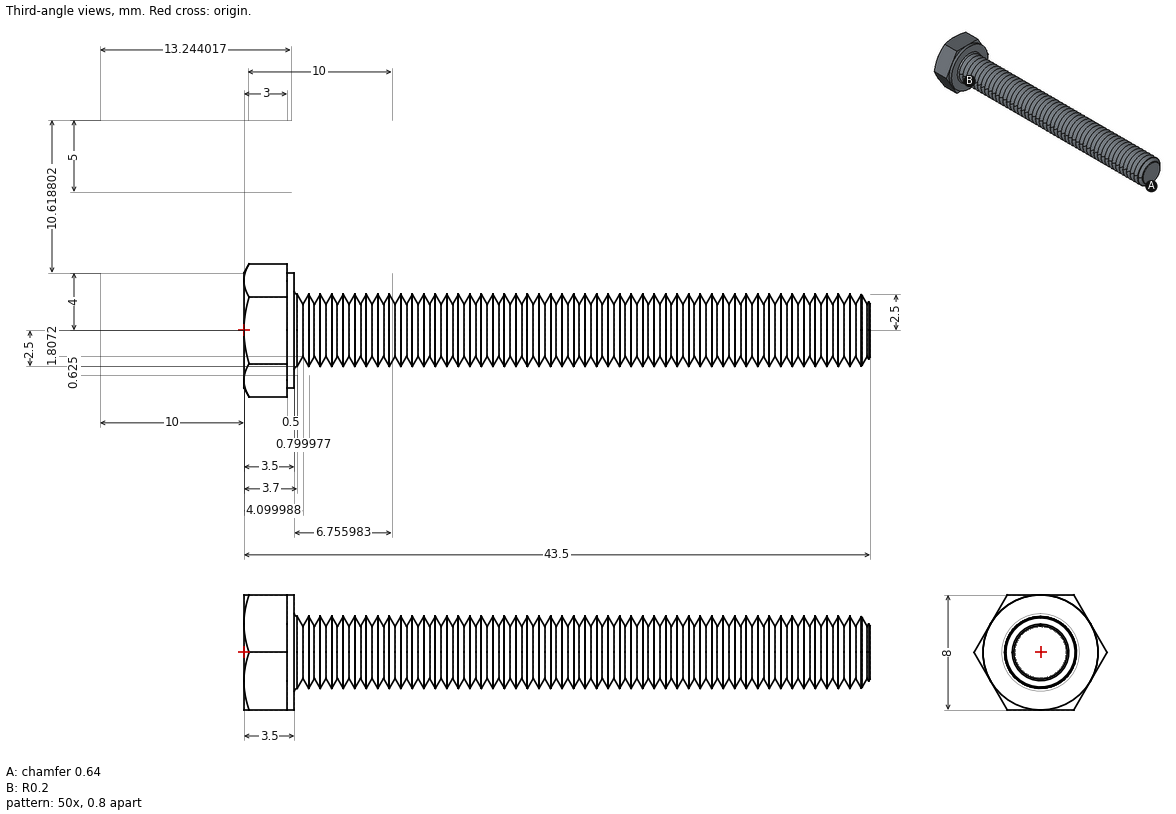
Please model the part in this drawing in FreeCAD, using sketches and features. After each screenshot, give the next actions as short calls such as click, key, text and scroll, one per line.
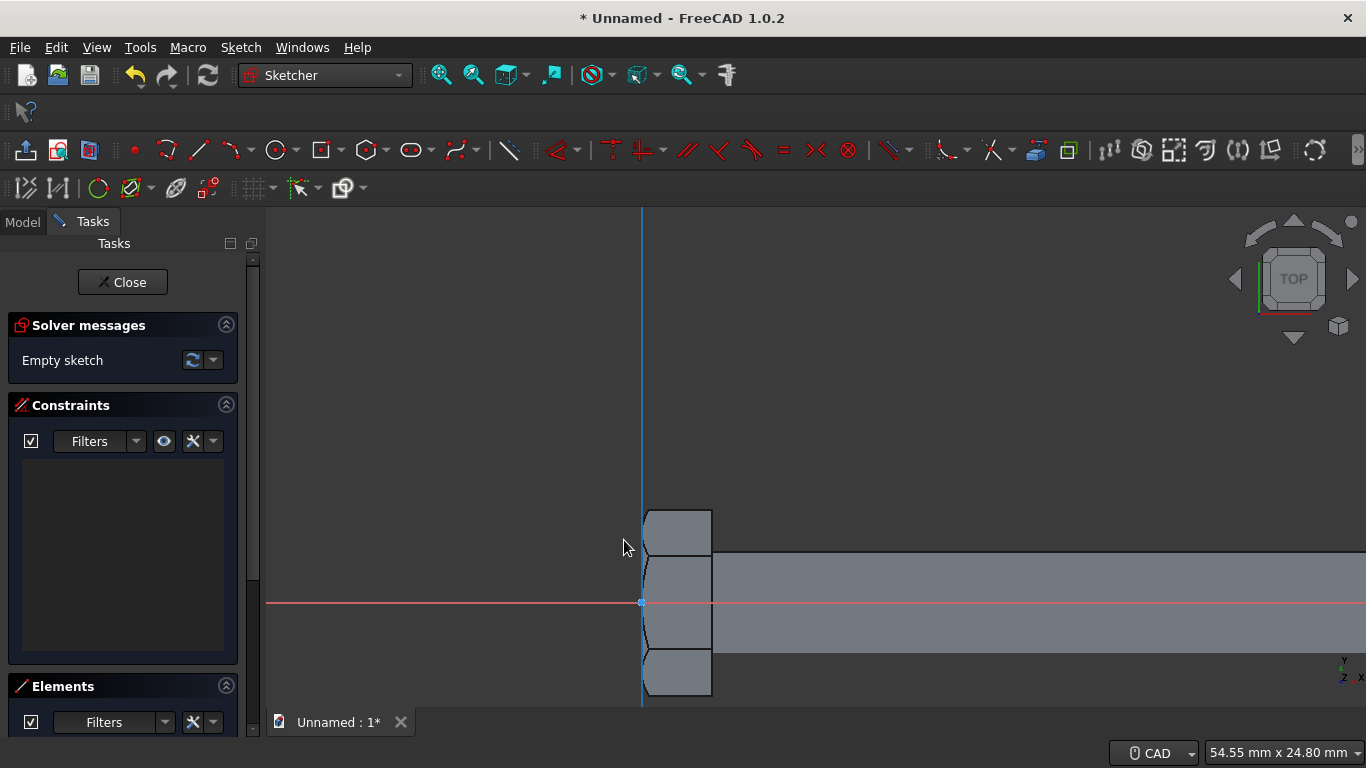
click(168, 150)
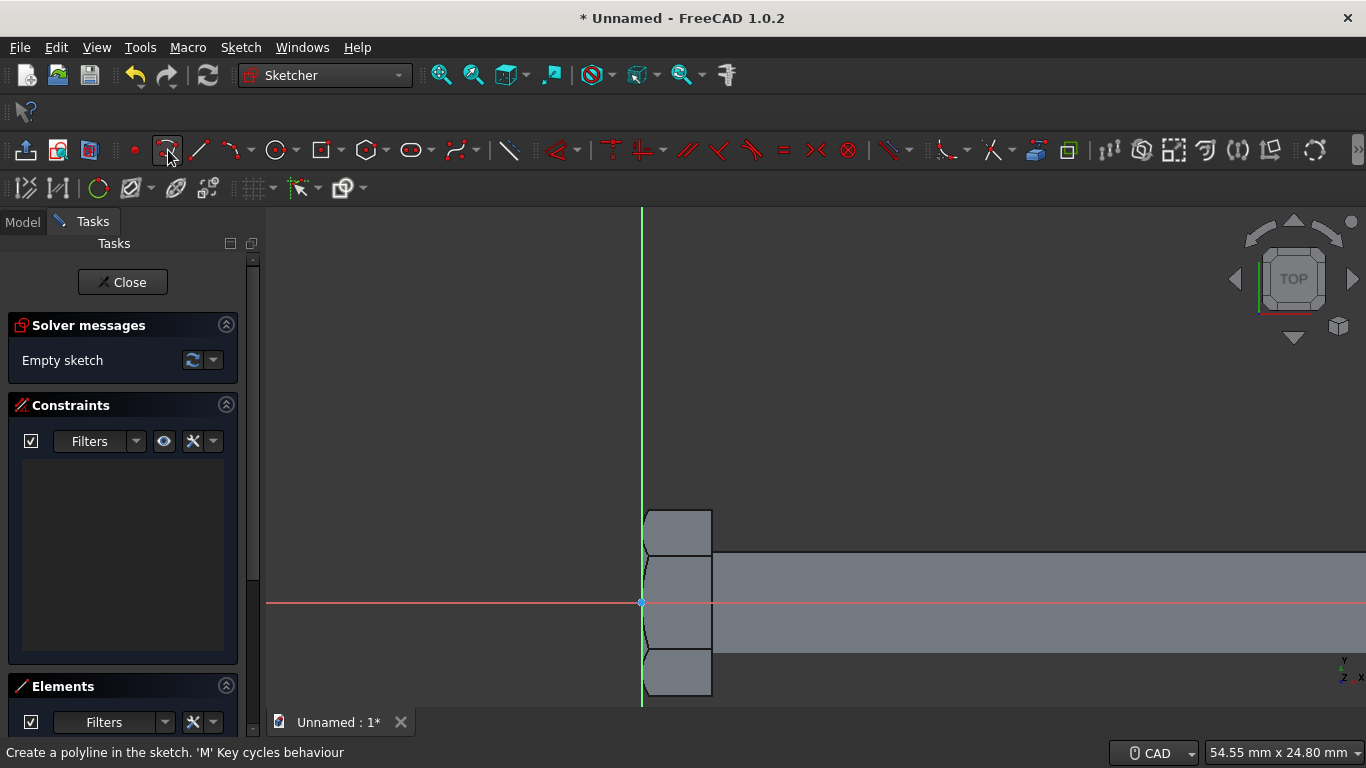
click(712, 522)
click(848, 522)
click(848, 308)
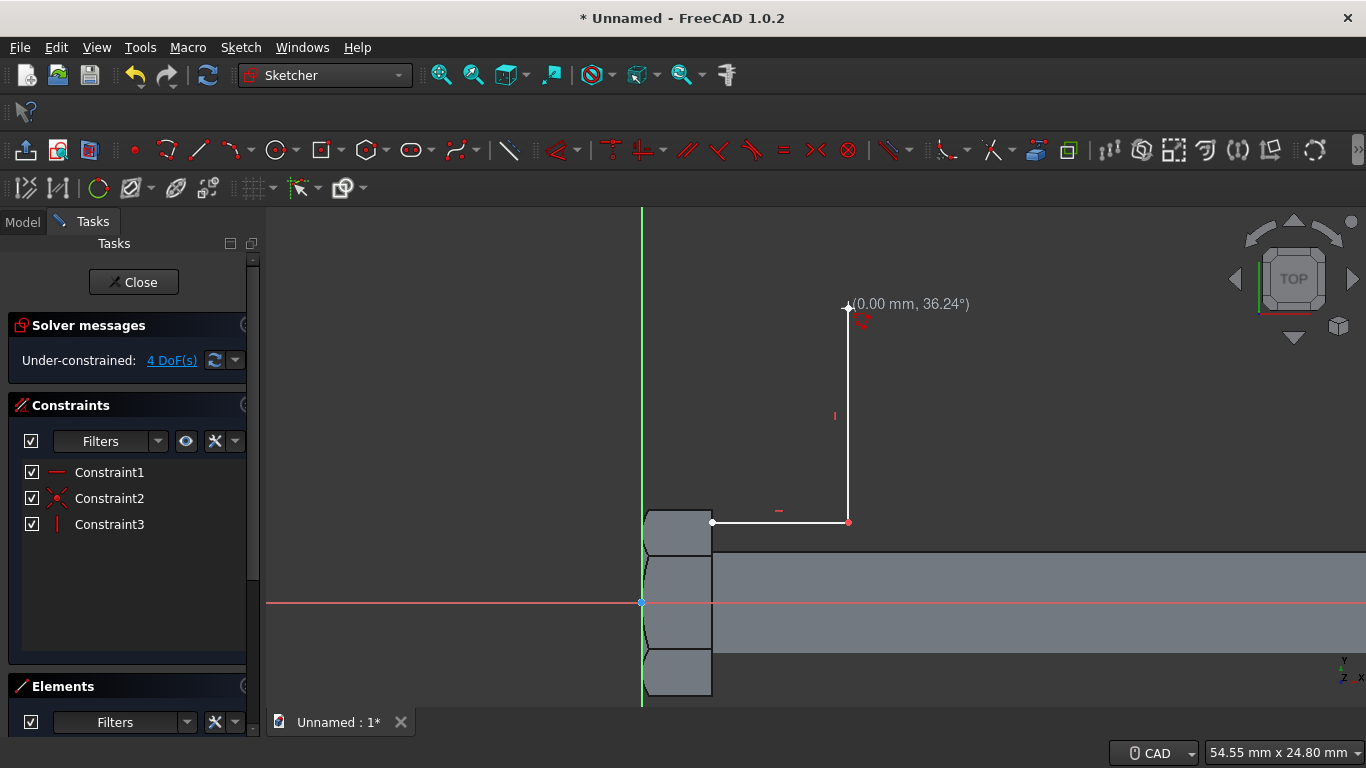
scroll(647, 308, up, 6)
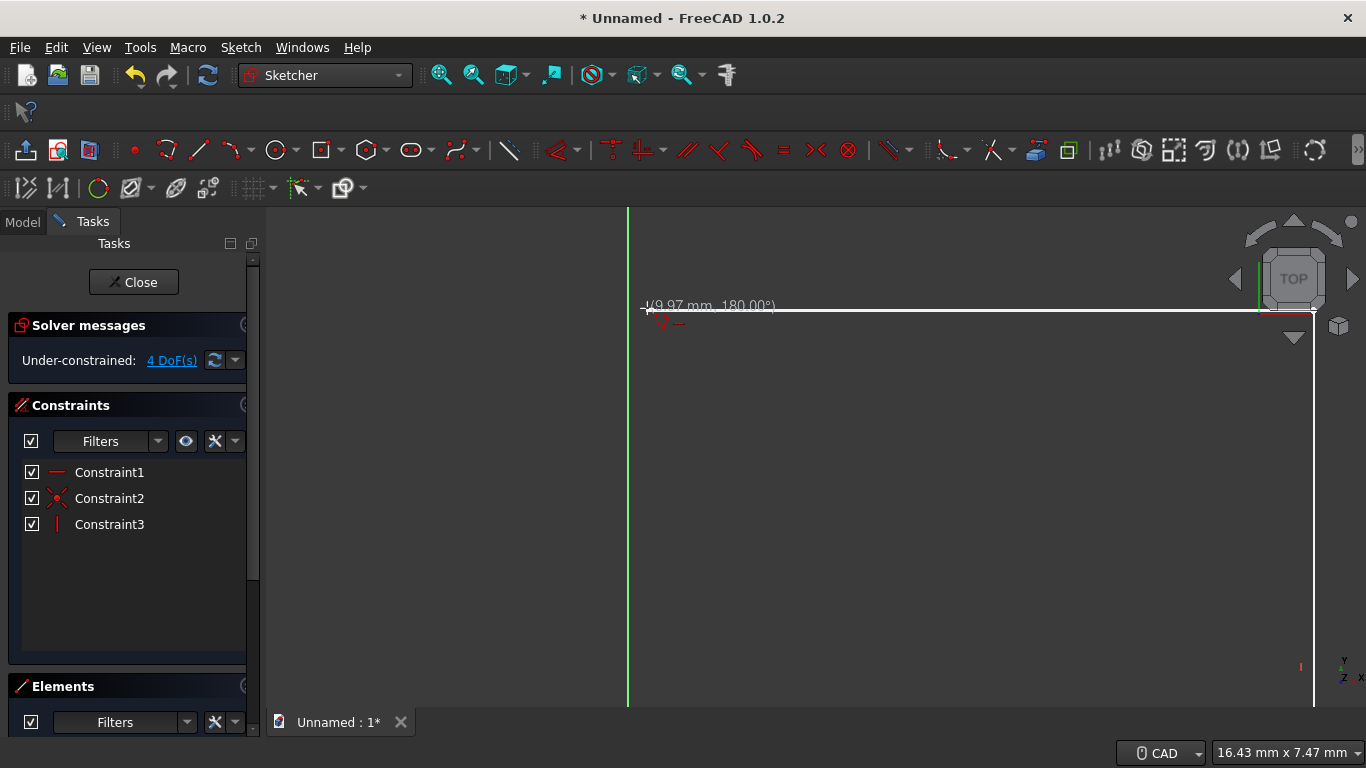
click(646, 308)
click(646, 642)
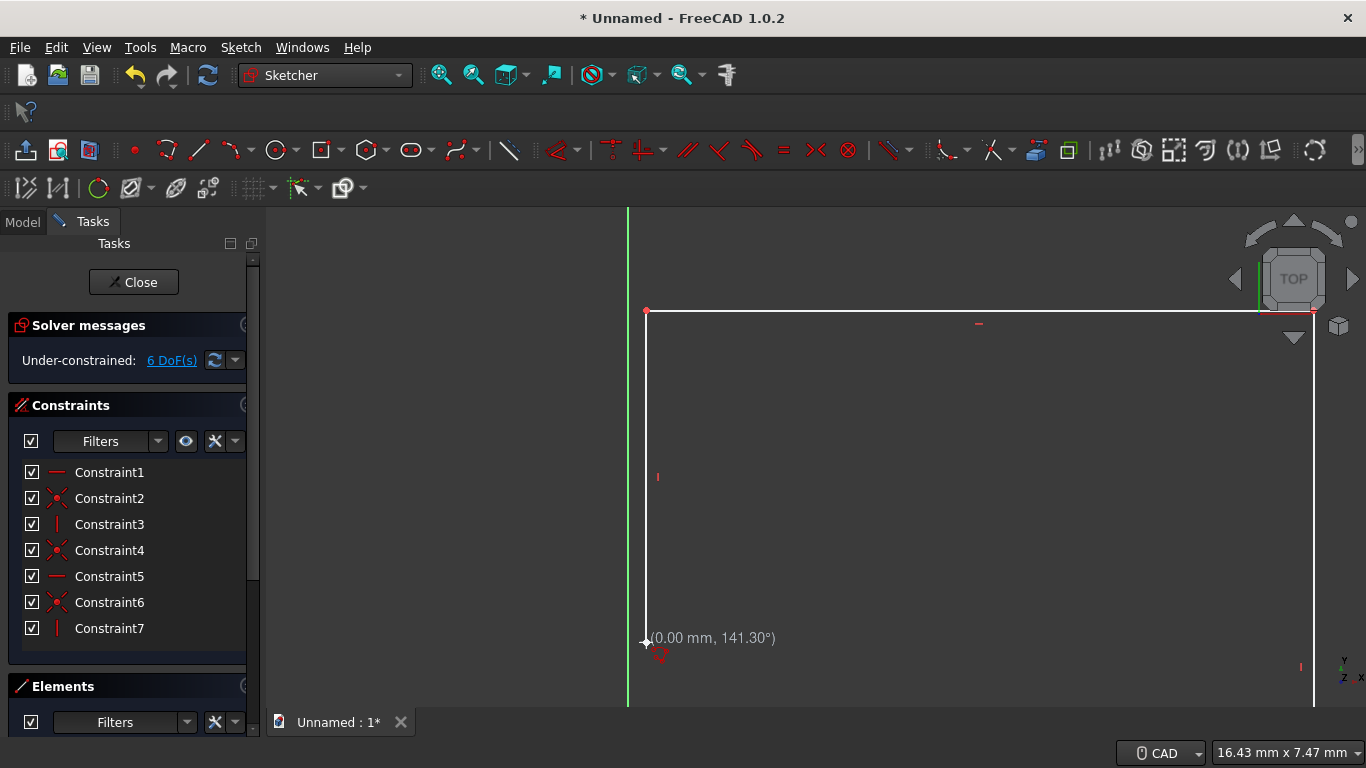
scroll(651, 311, down, 6)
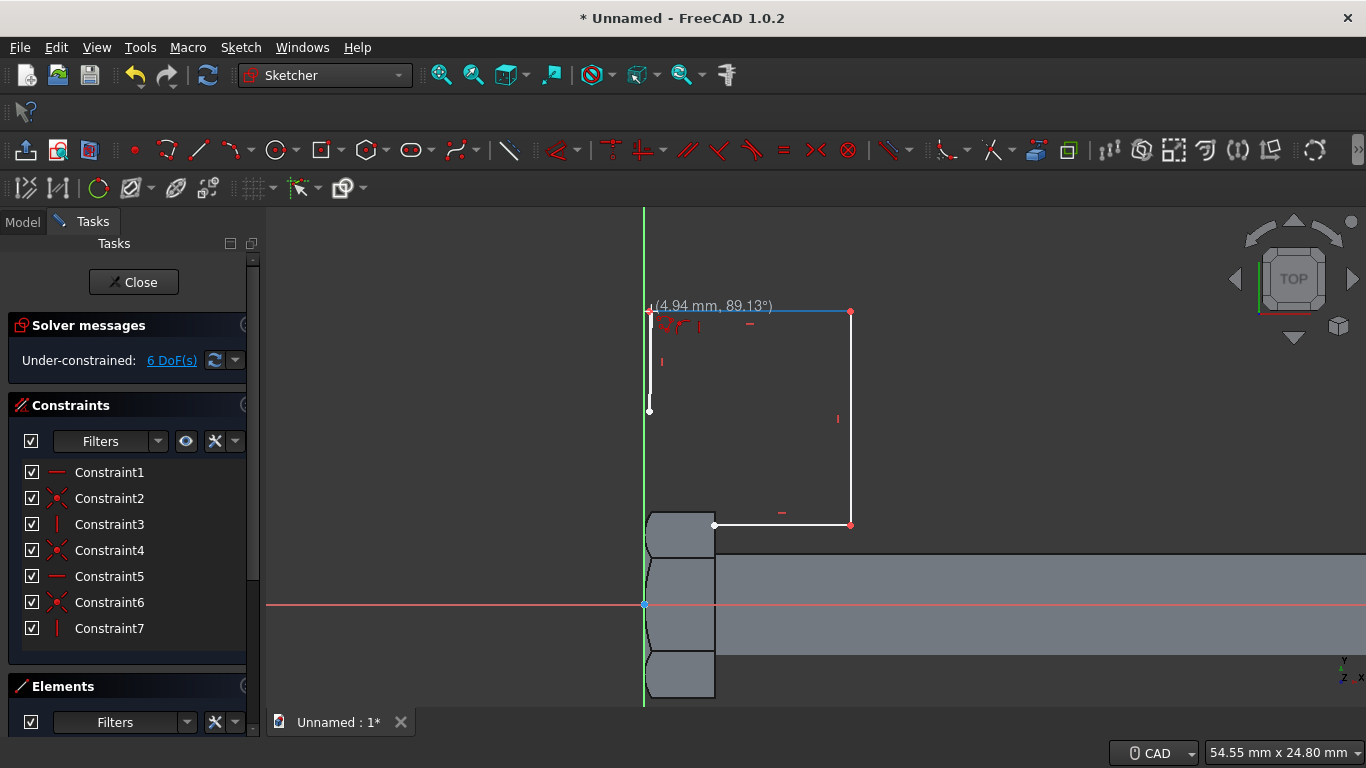
click(715, 525)
key(Escape)
key(Escape)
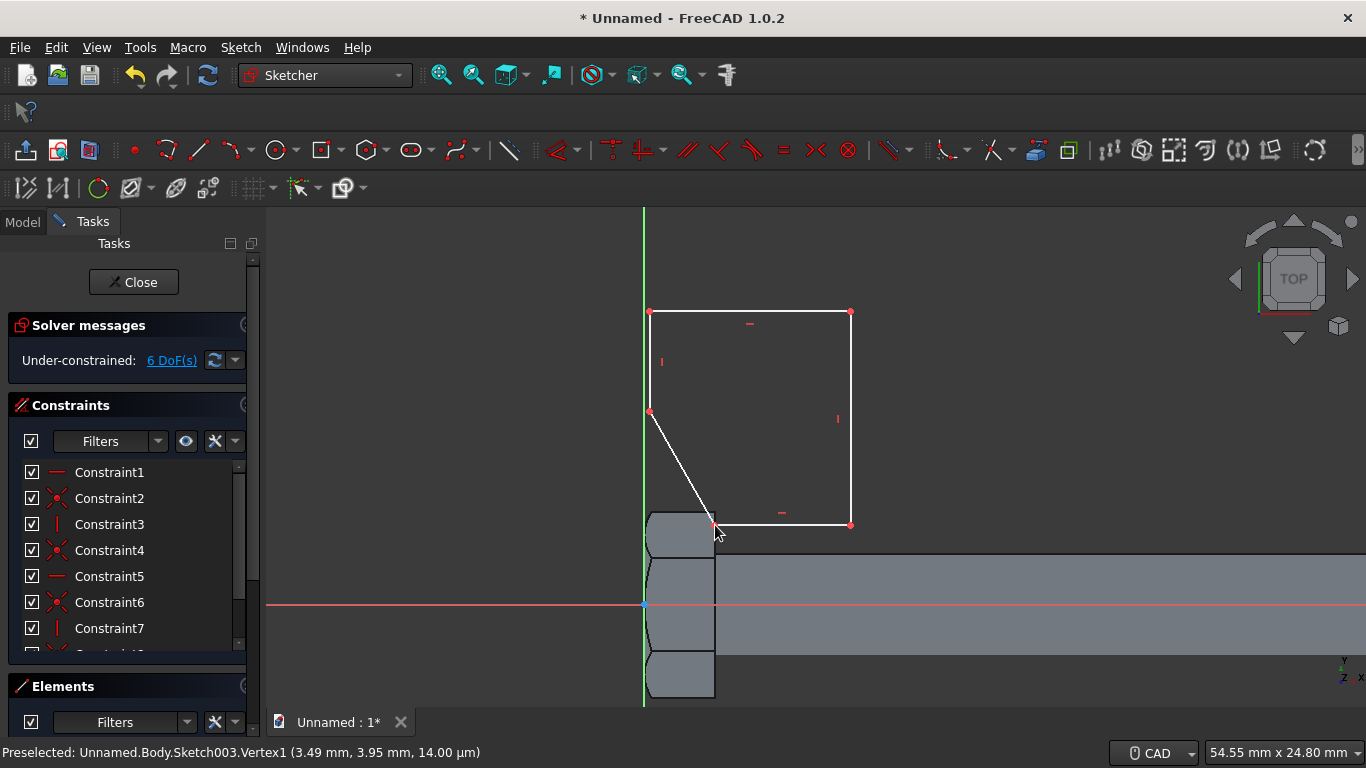
click(556, 150)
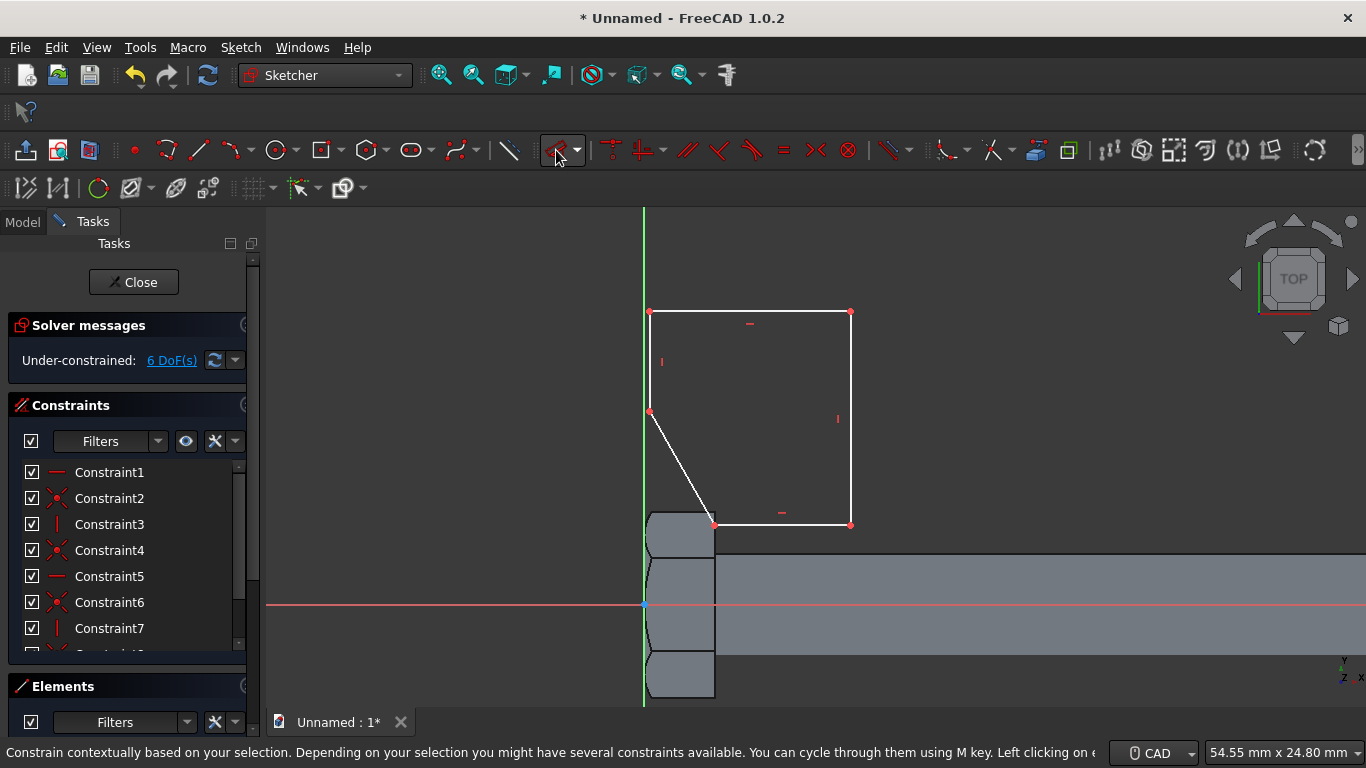
scroll(650, 341, up, 5)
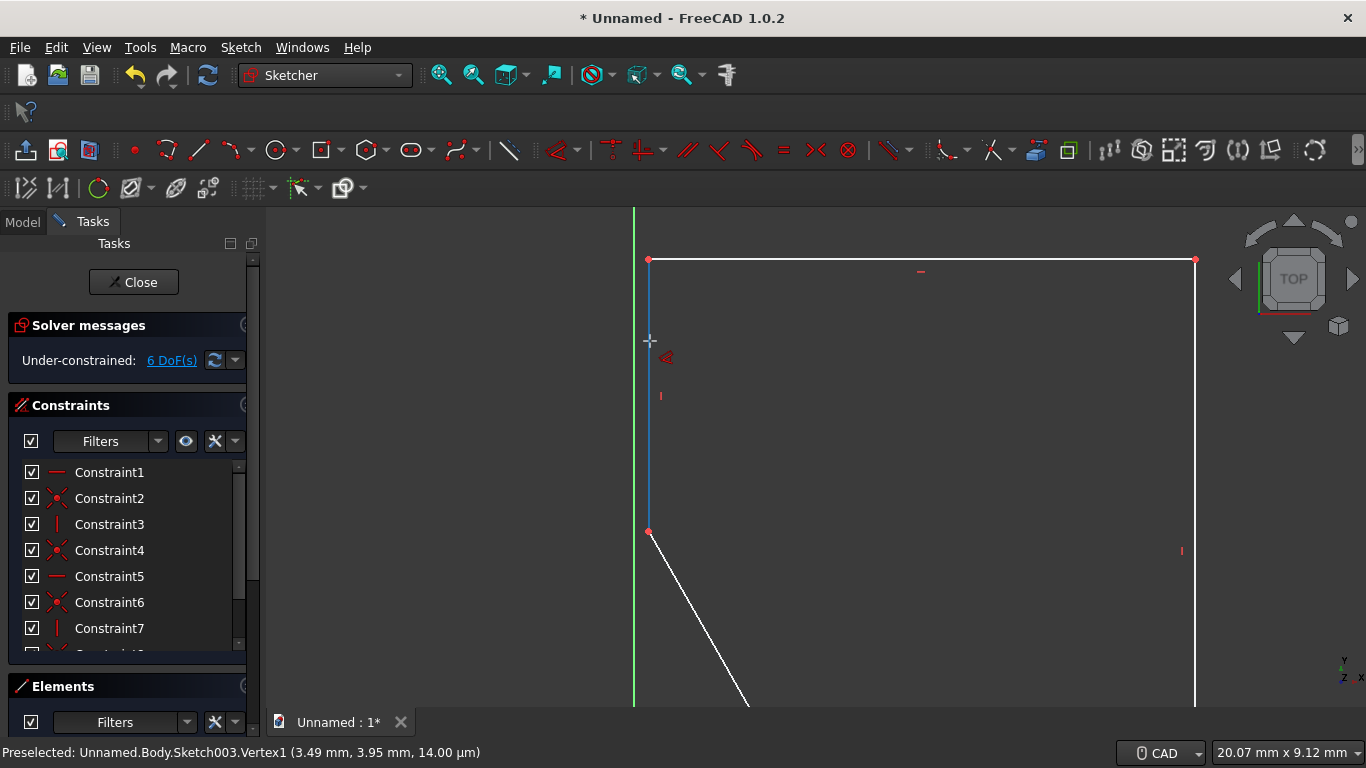
click(649, 341)
click(615, 395)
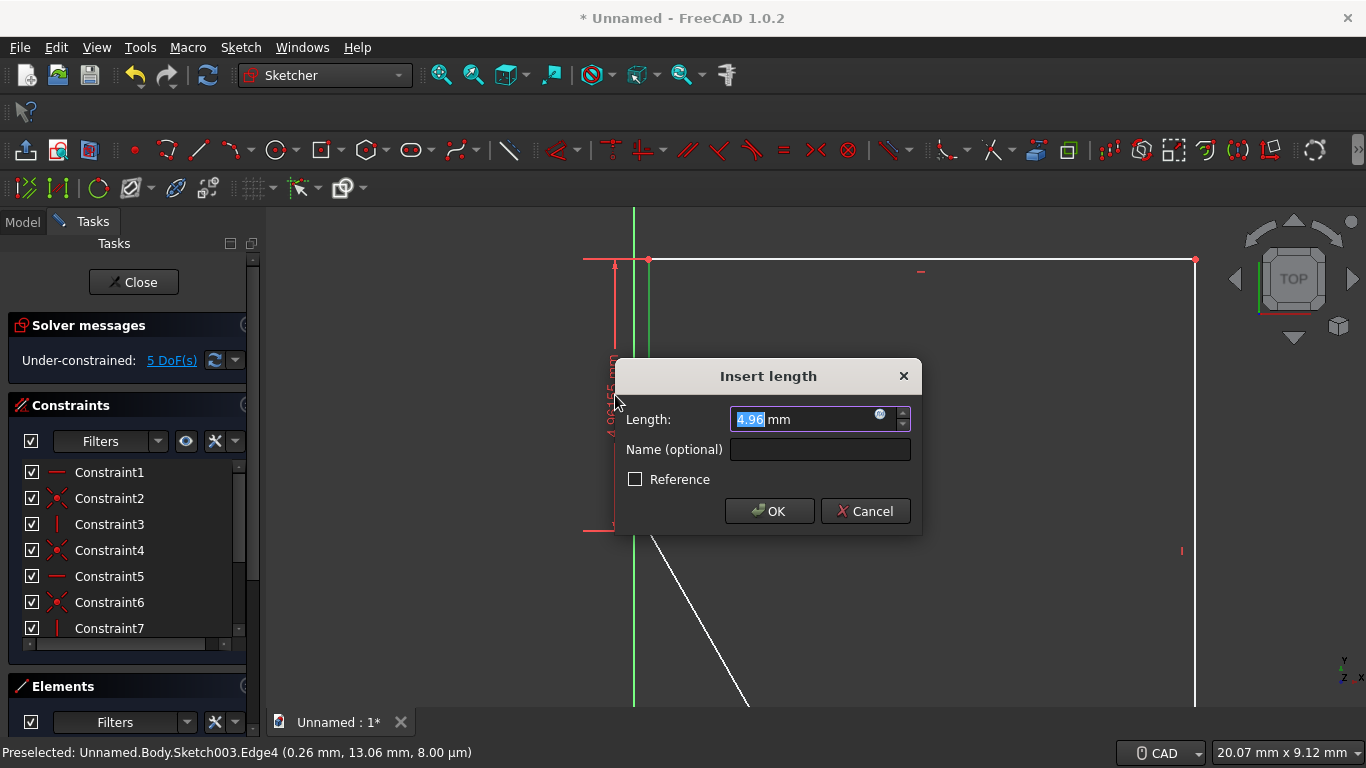
text(5)
key(Return)